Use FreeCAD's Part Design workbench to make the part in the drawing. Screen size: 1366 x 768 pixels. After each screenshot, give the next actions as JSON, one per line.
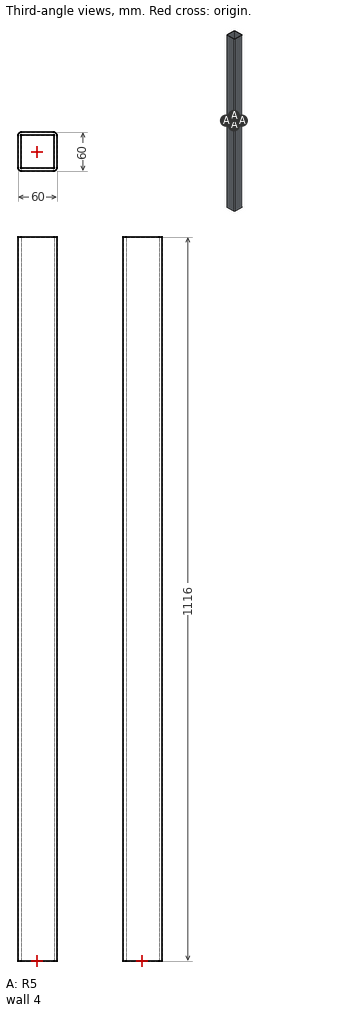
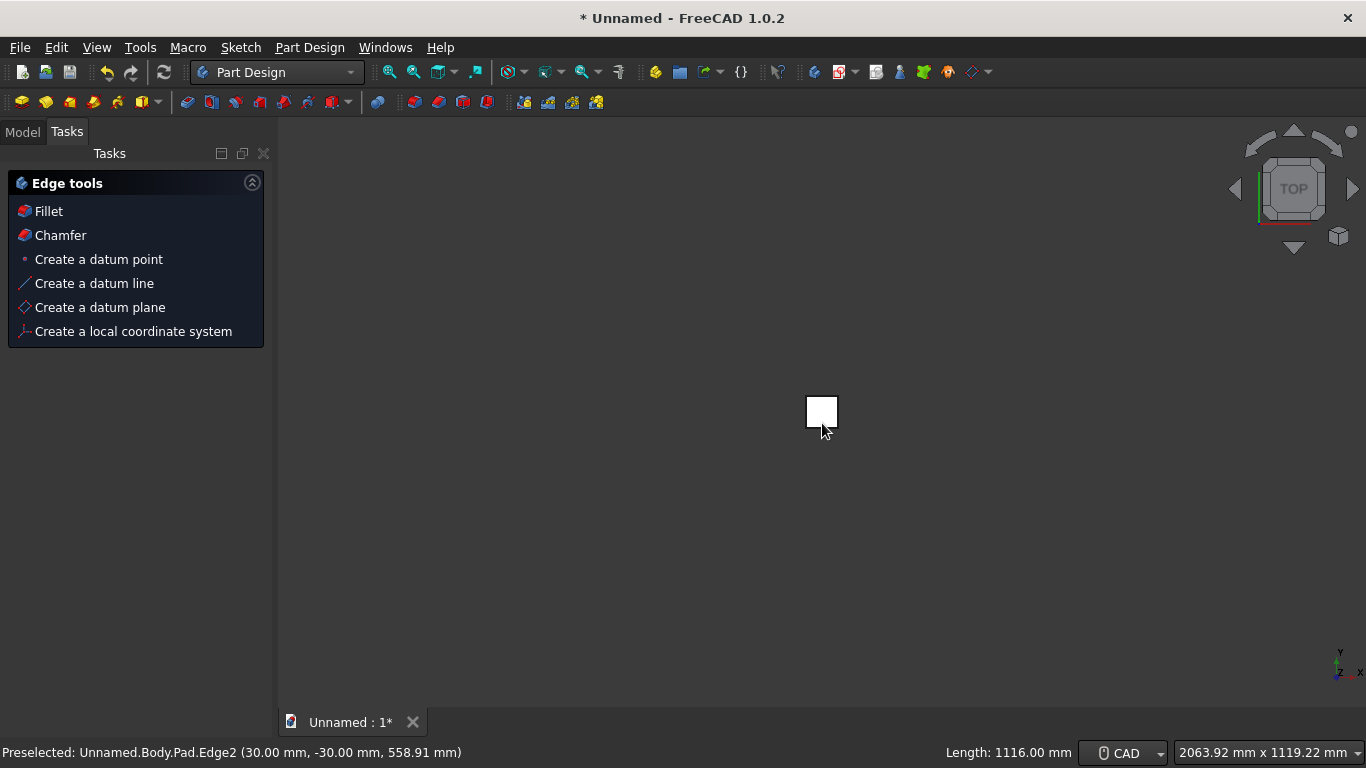
{"action": "left_click", "coordinate": [390, 72]}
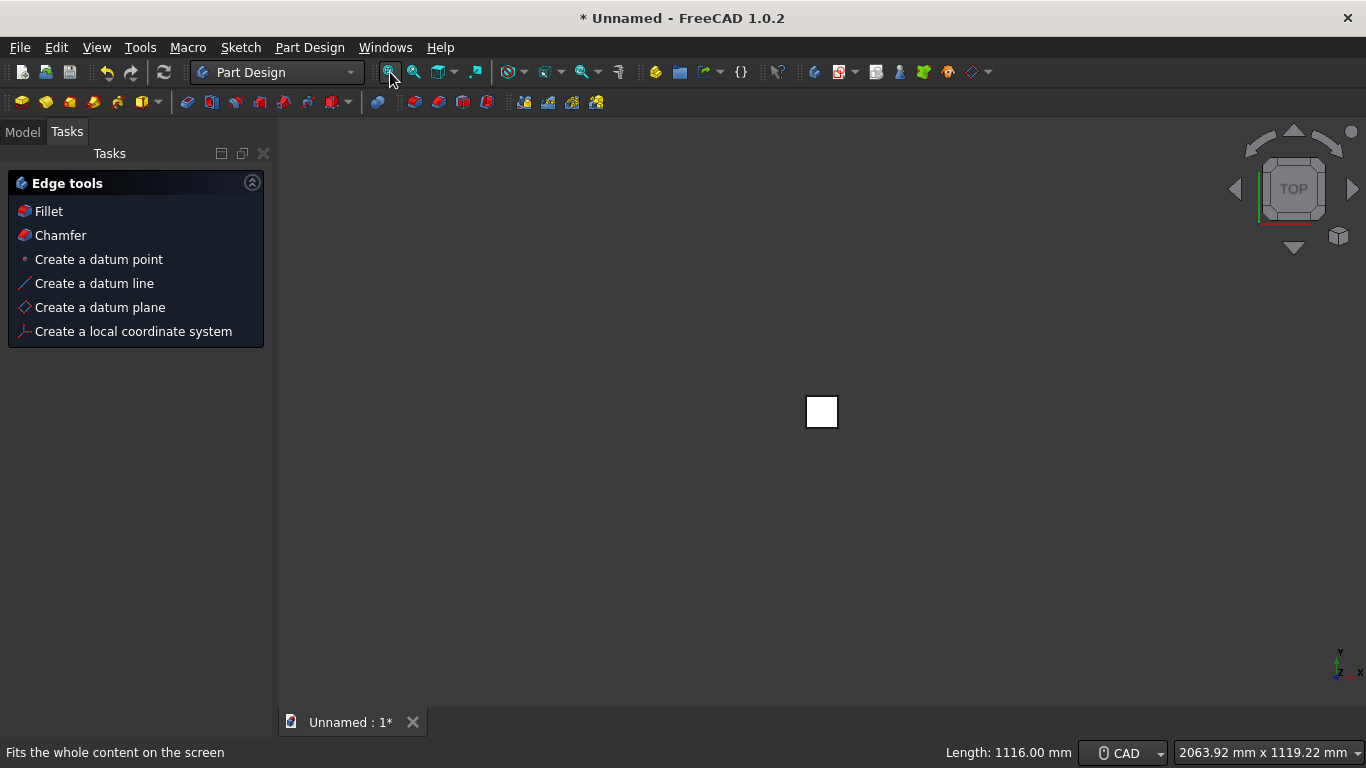
{"action": "key", "text": "1"}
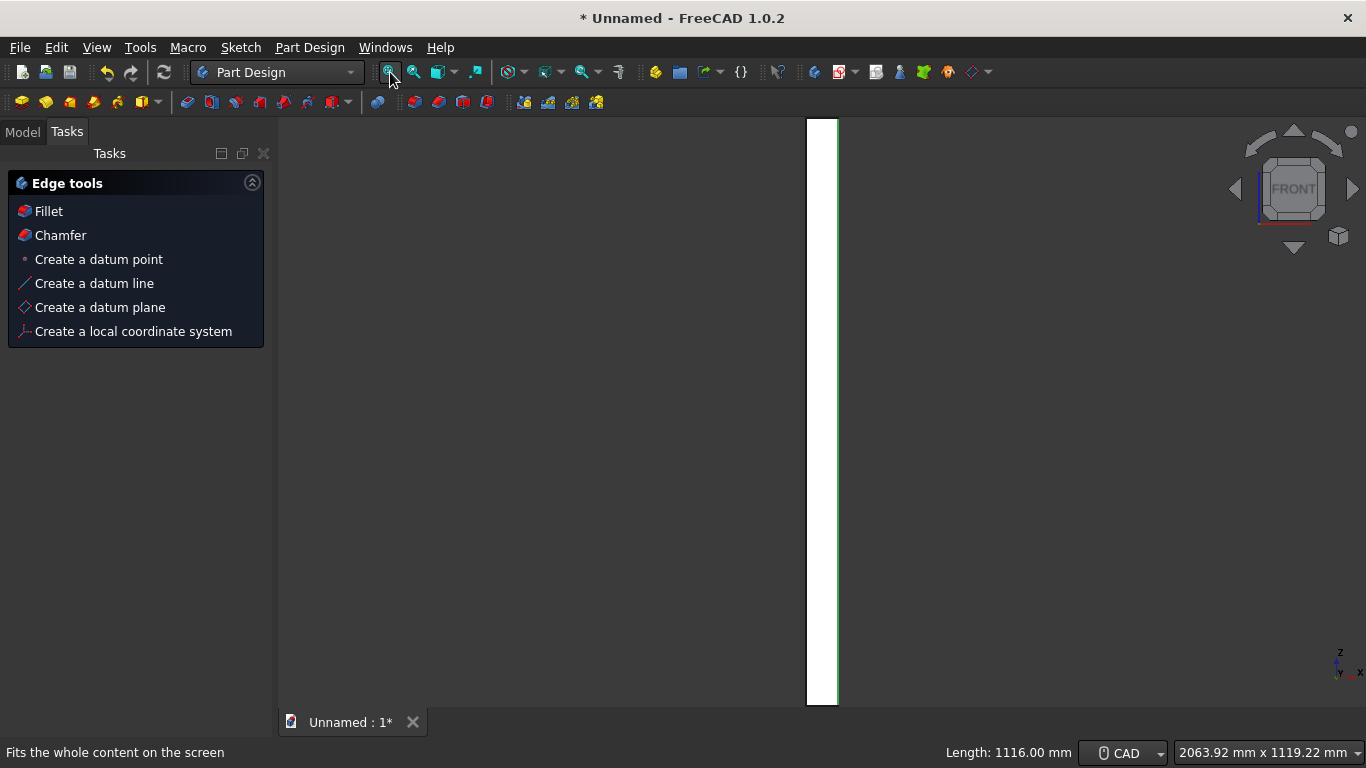
{"action": "left_click", "coordinate": [806, 411], "text": "ctrl"}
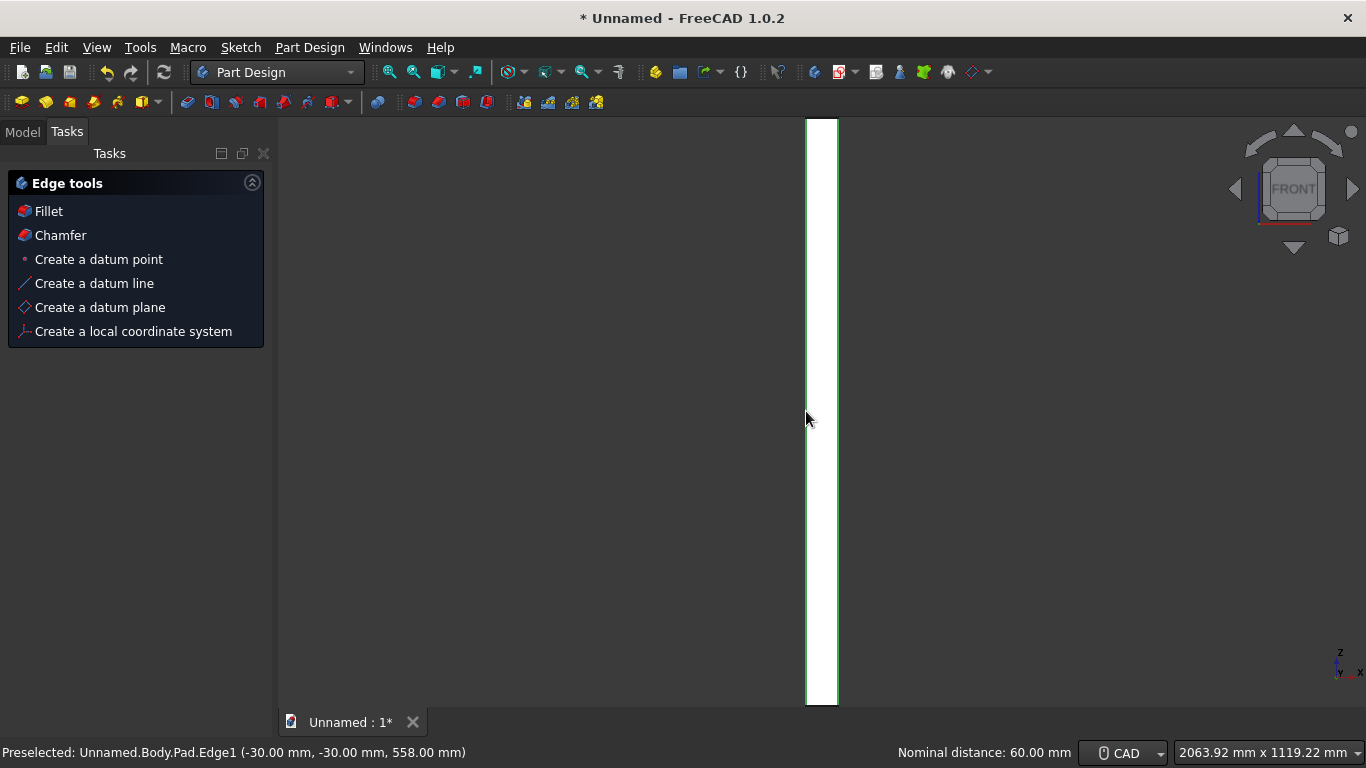
{"action": "key", "text": "3"}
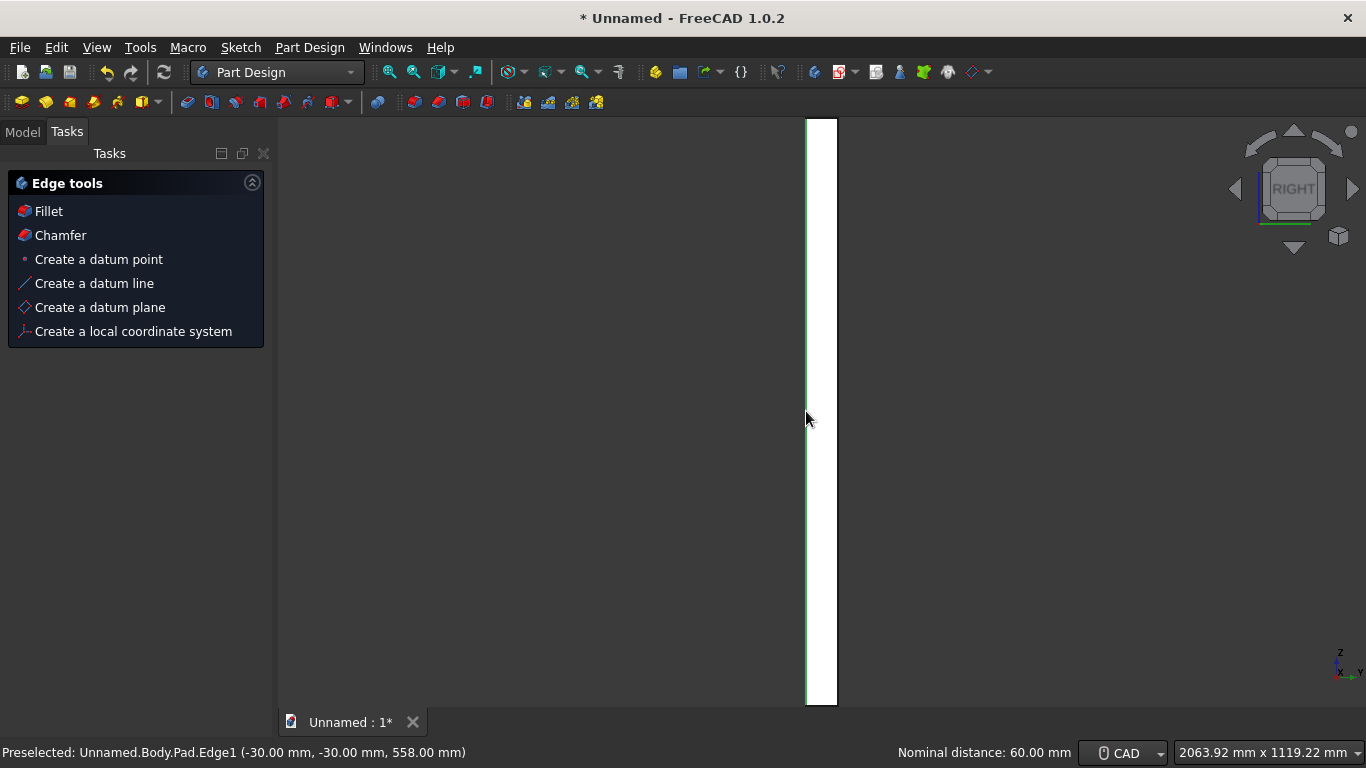
{"action": "left_click", "coordinate": [838, 411], "text": "ctrl"}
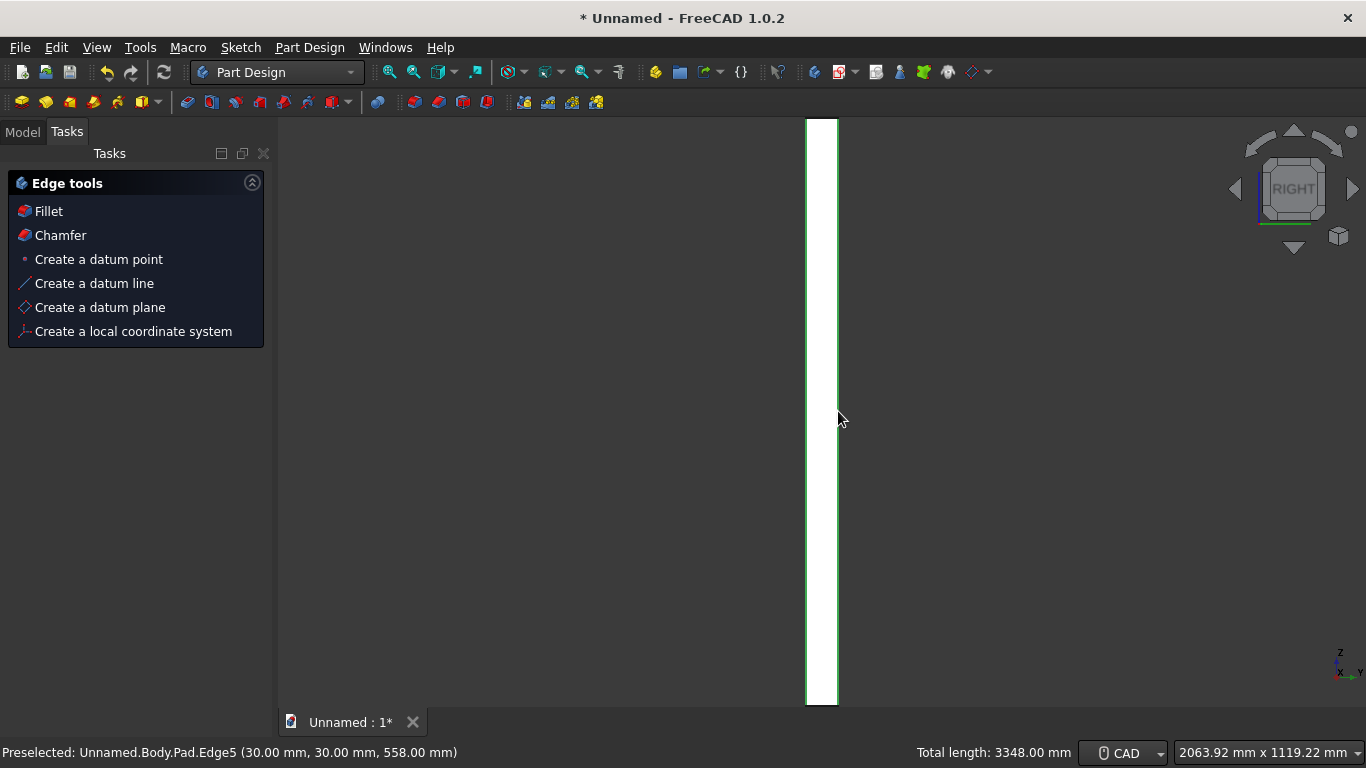
{"action": "key", "text": "5"}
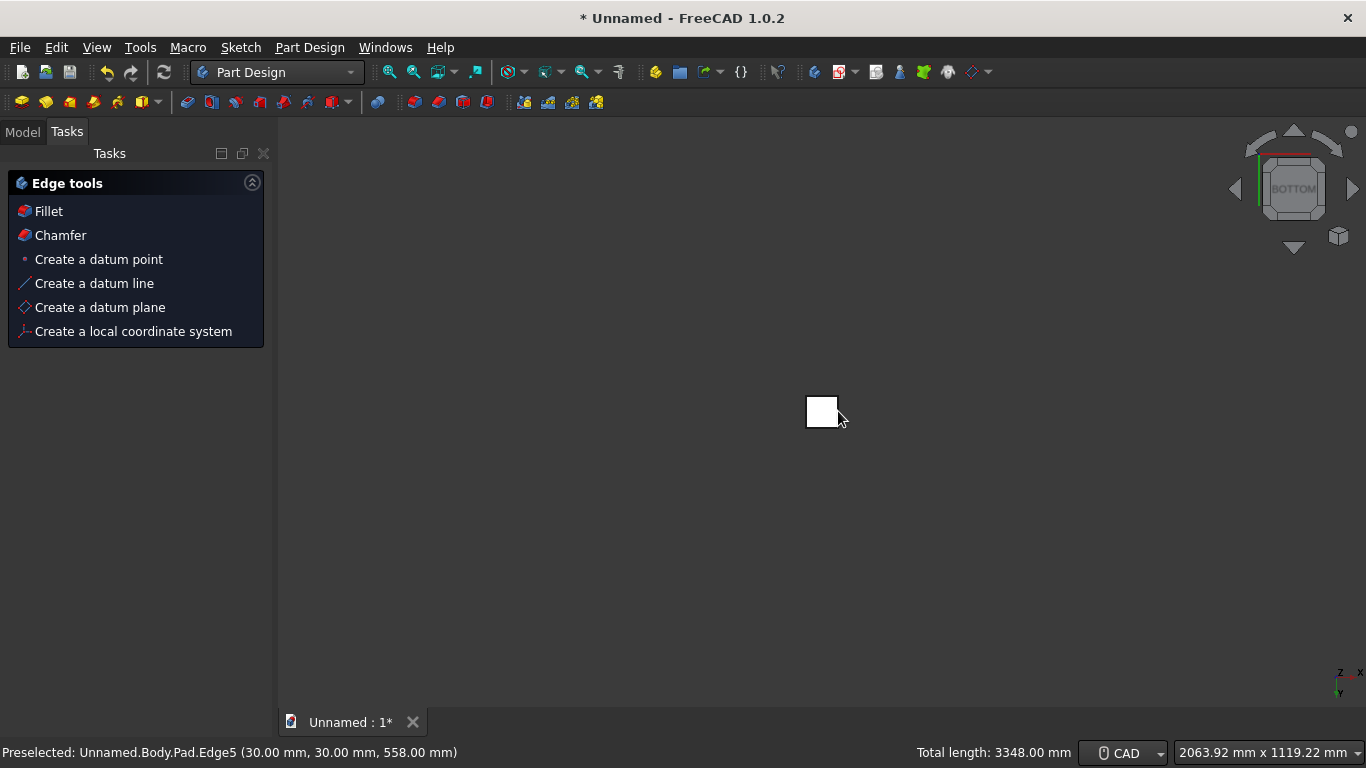
{"action": "key", "text": "v f"}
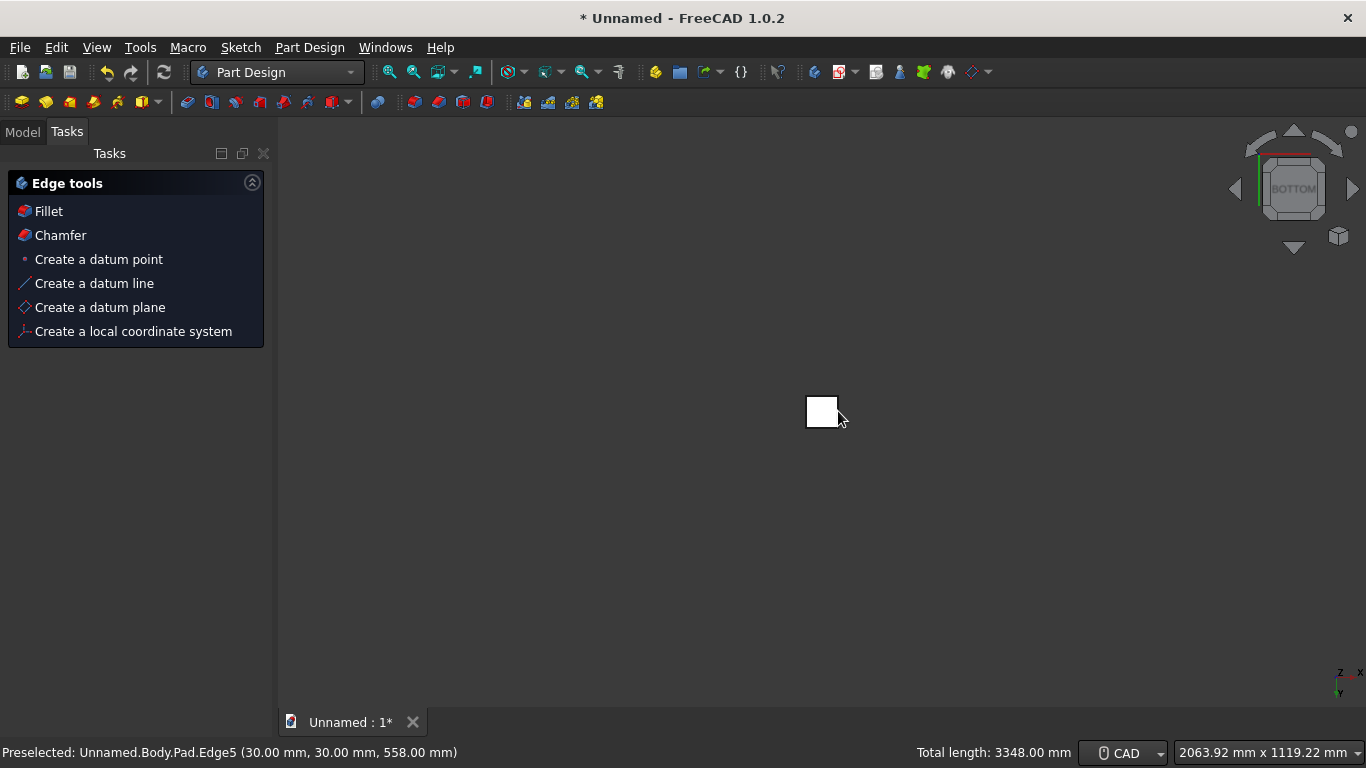
{"action": "key", "text": "4"}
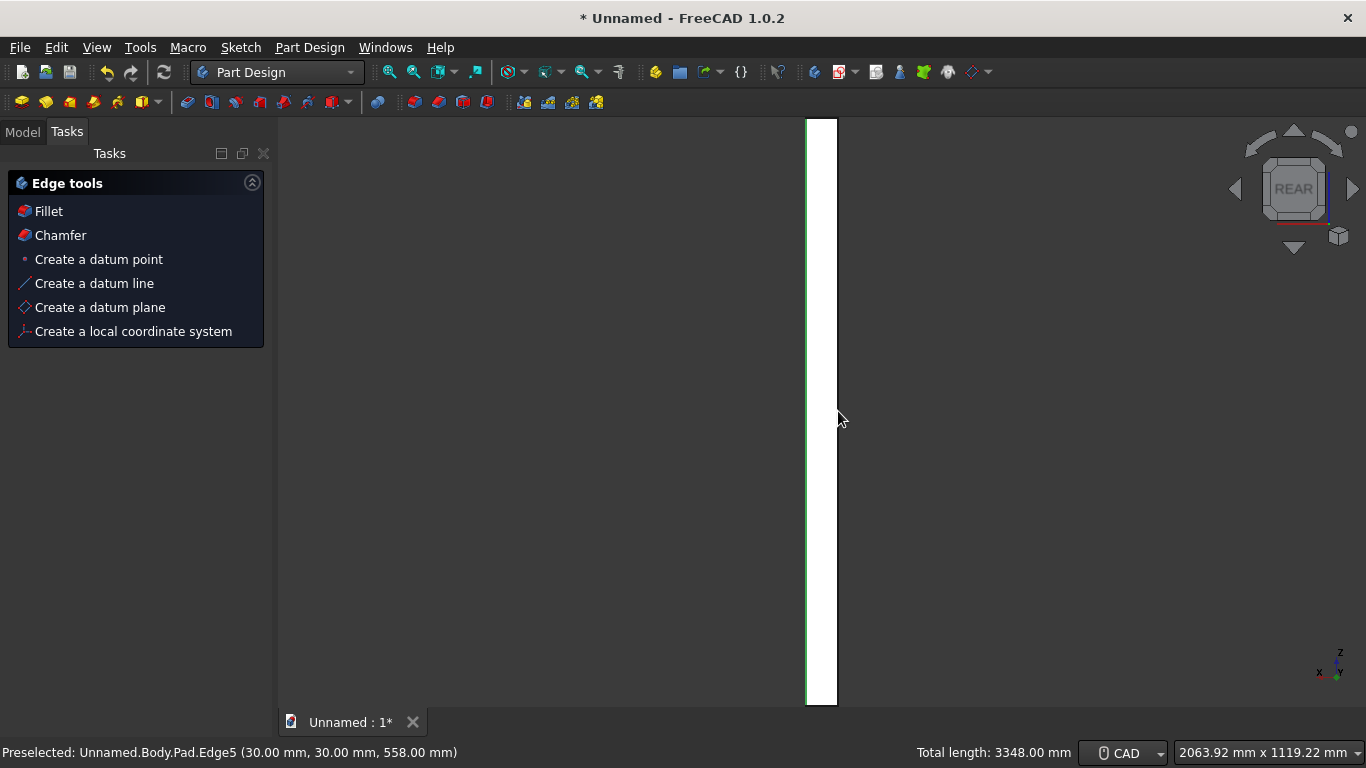
{"action": "left_click", "coordinate": [838, 411], "text": "ctrl"}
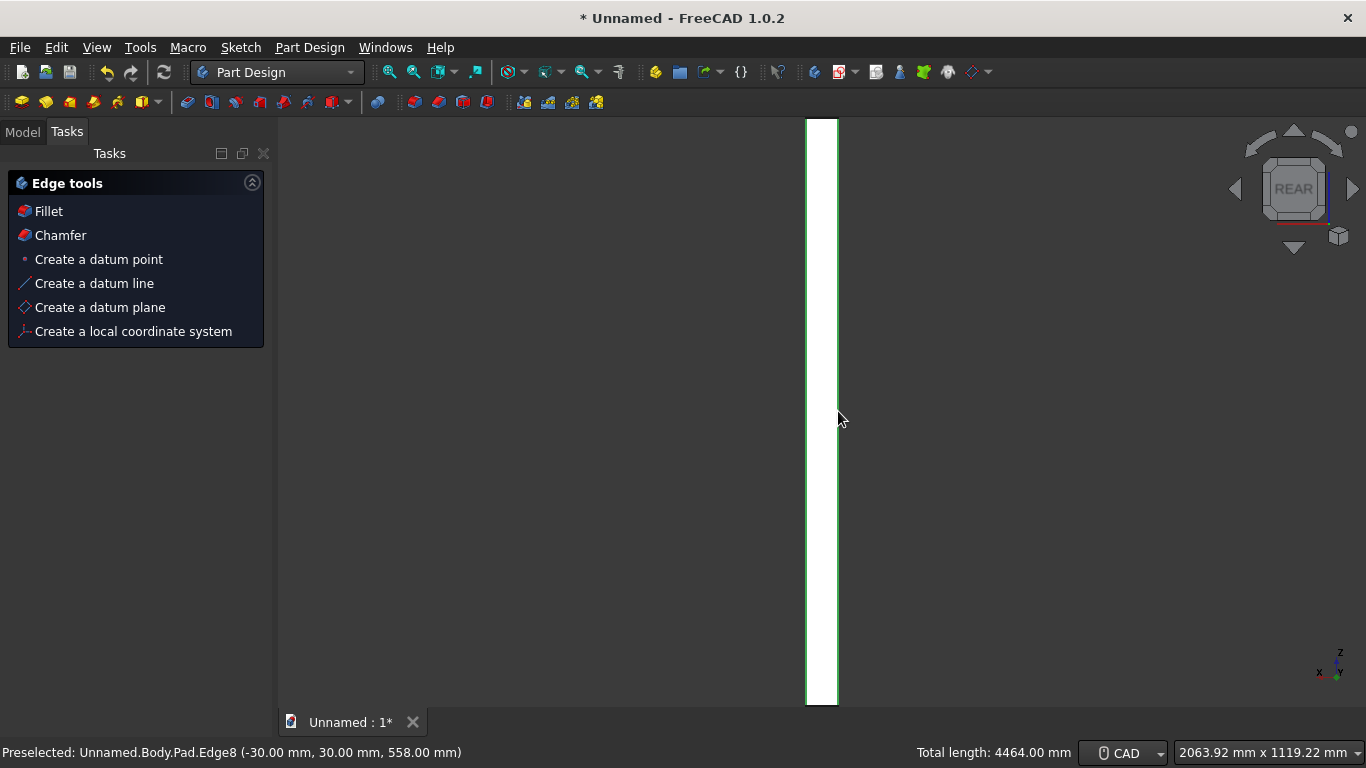
{"action": "left_click", "coordinate": [416, 102]}